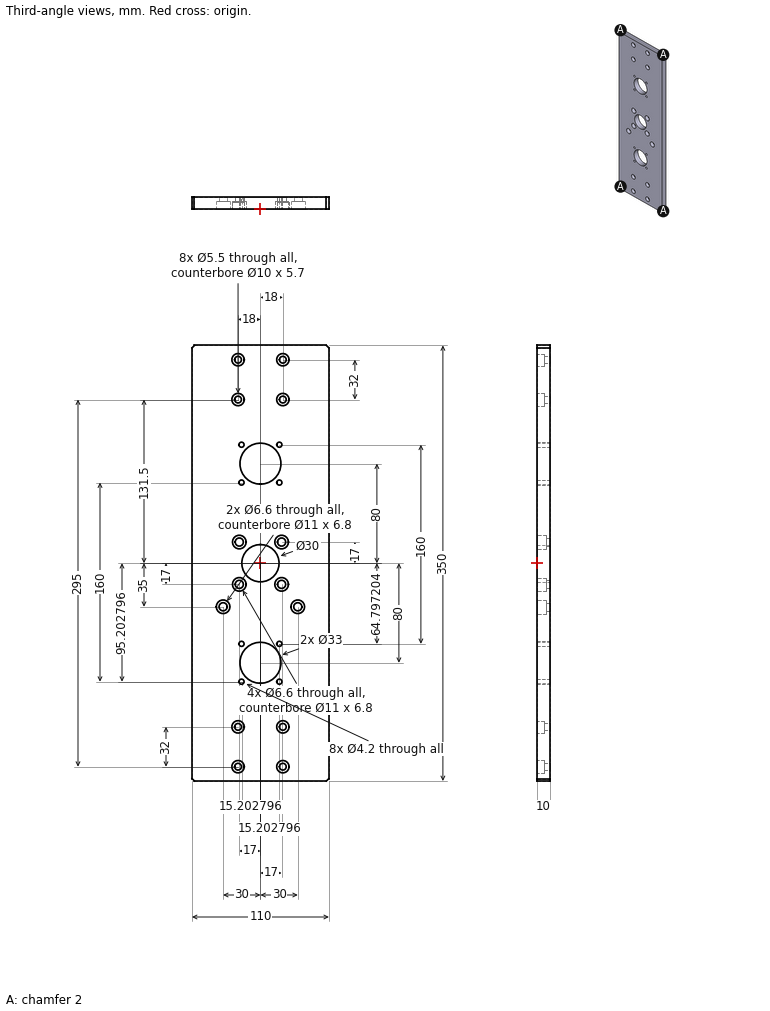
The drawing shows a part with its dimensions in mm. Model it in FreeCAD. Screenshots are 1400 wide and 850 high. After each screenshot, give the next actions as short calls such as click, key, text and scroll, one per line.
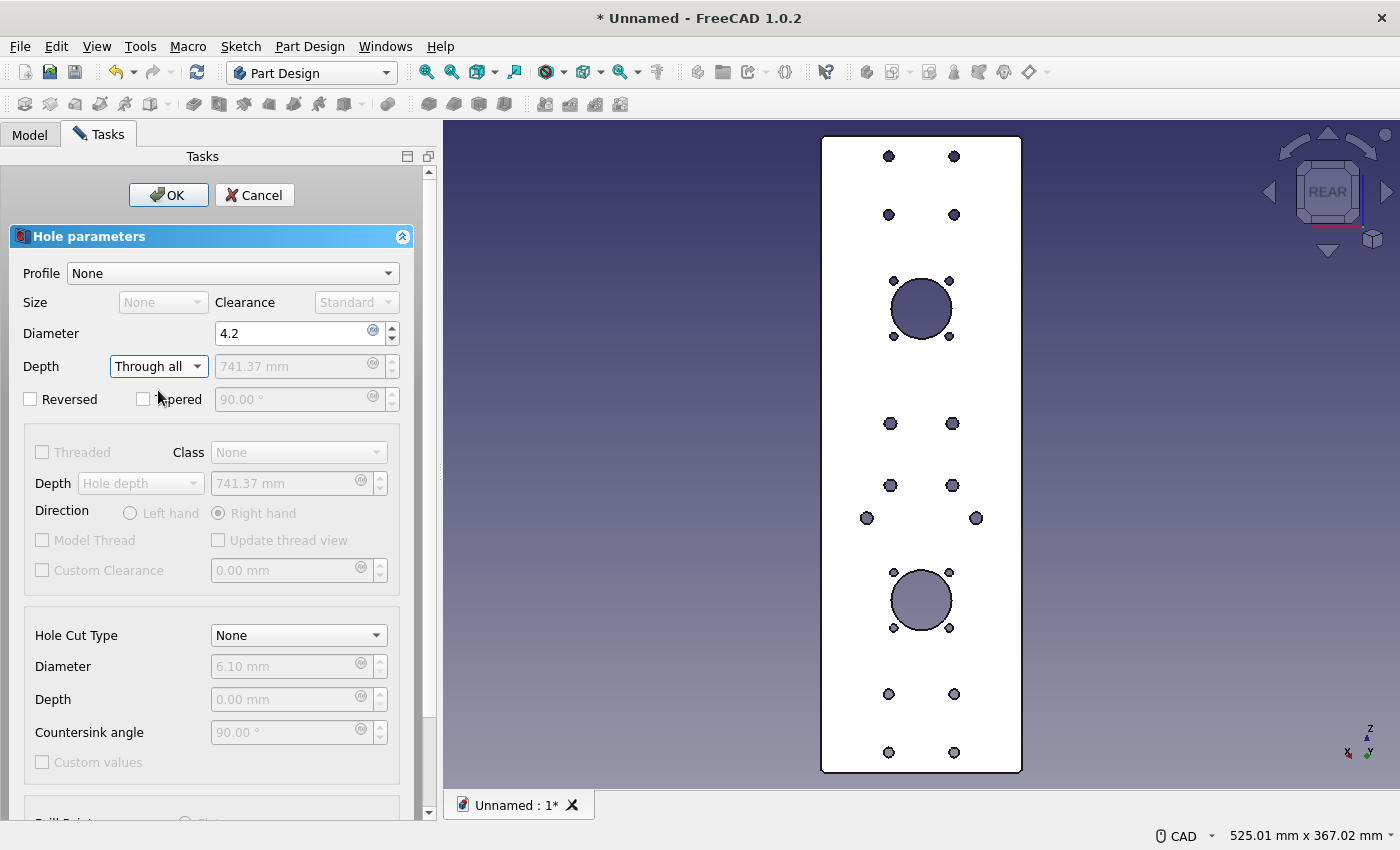
click(169, 195)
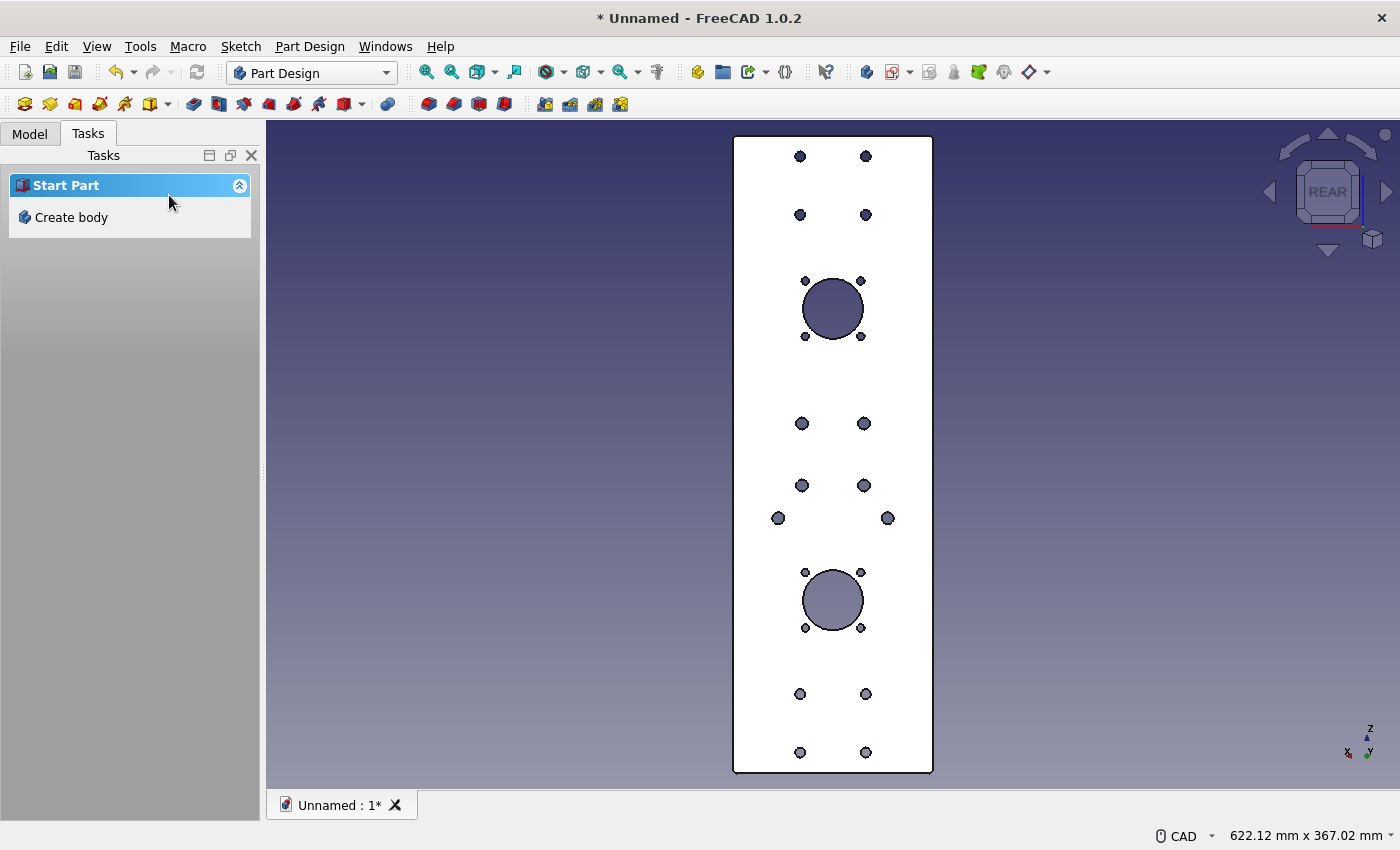
click(833, 454)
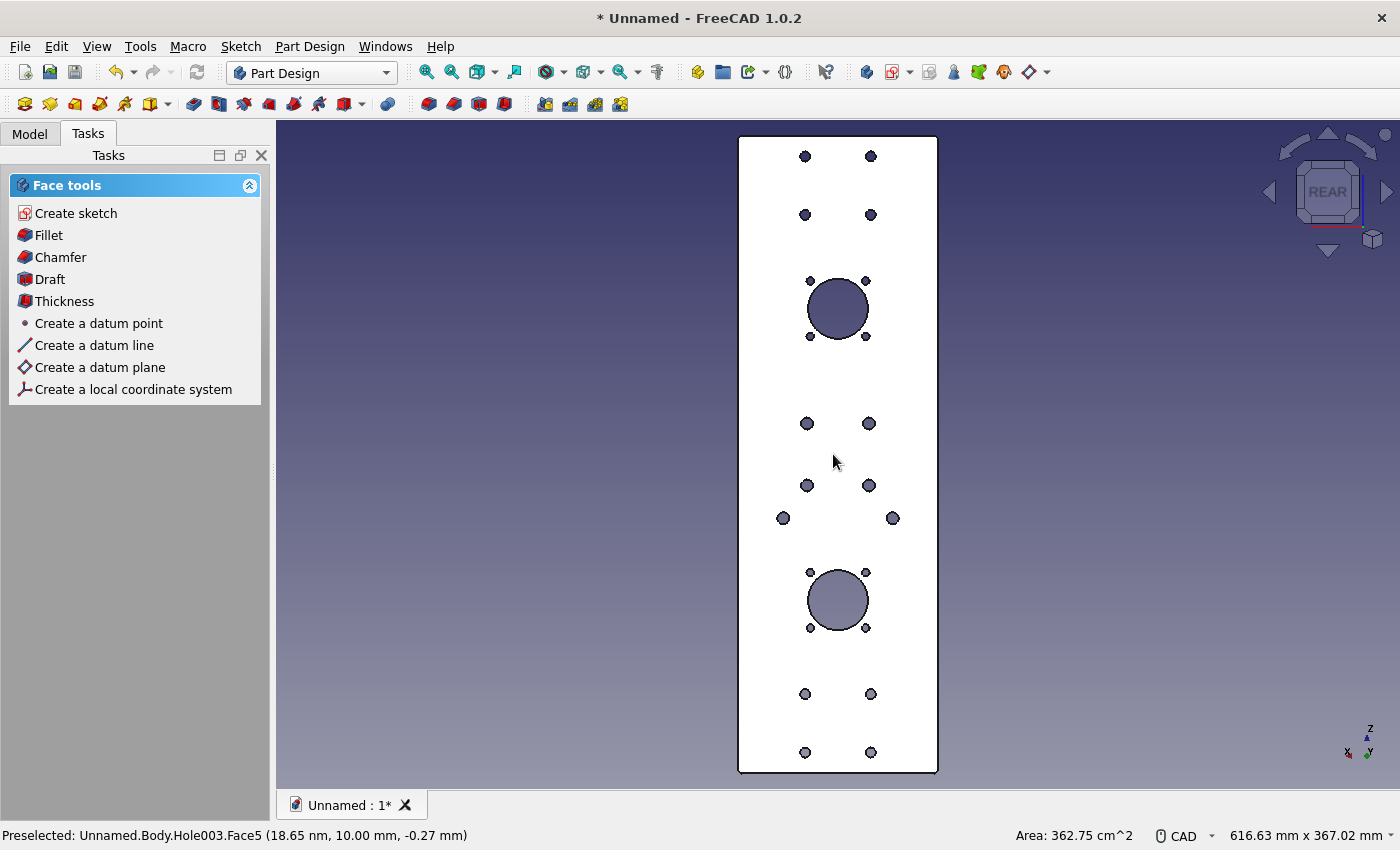
click(892, 72)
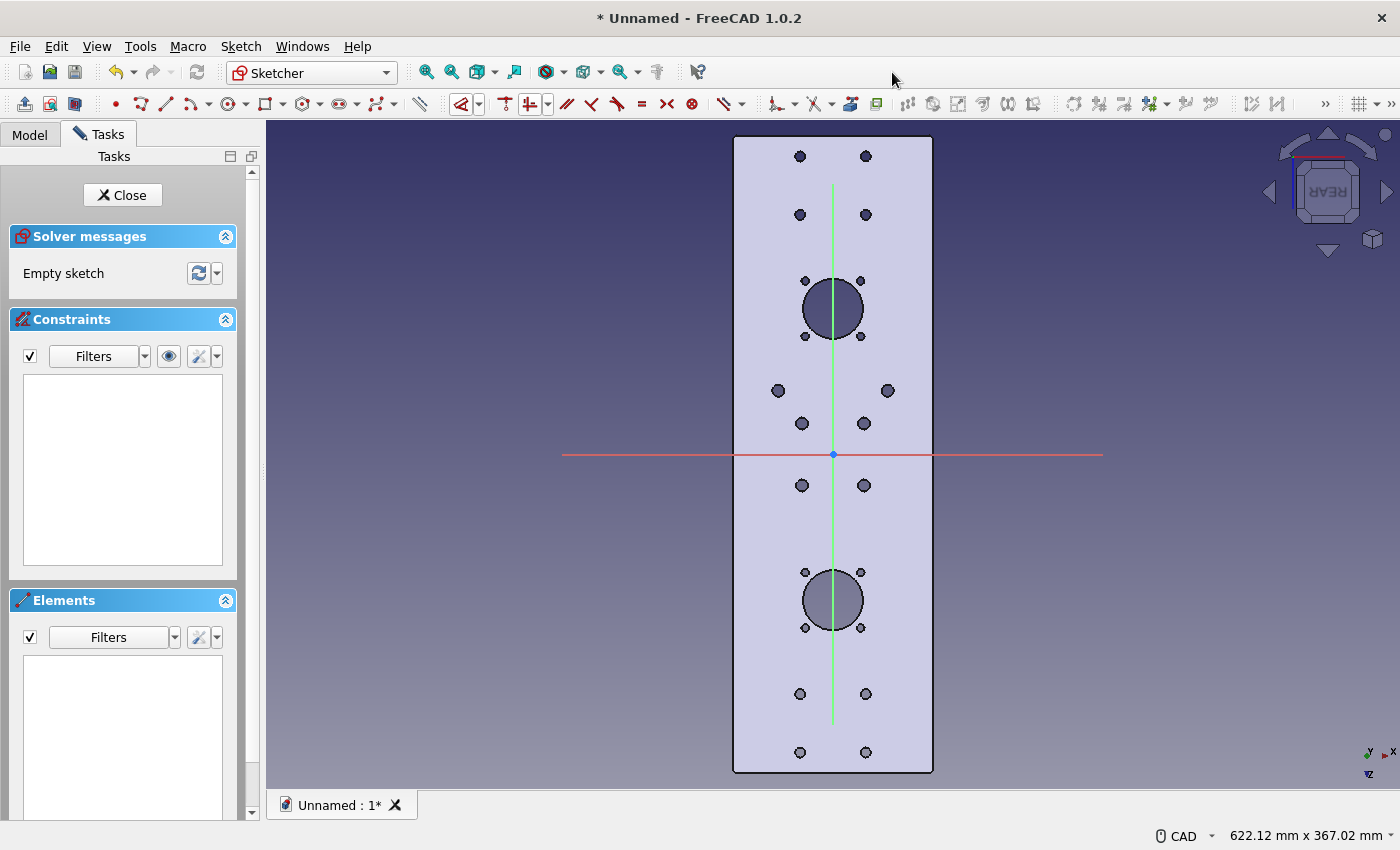
scroll(844, 454, up, 10)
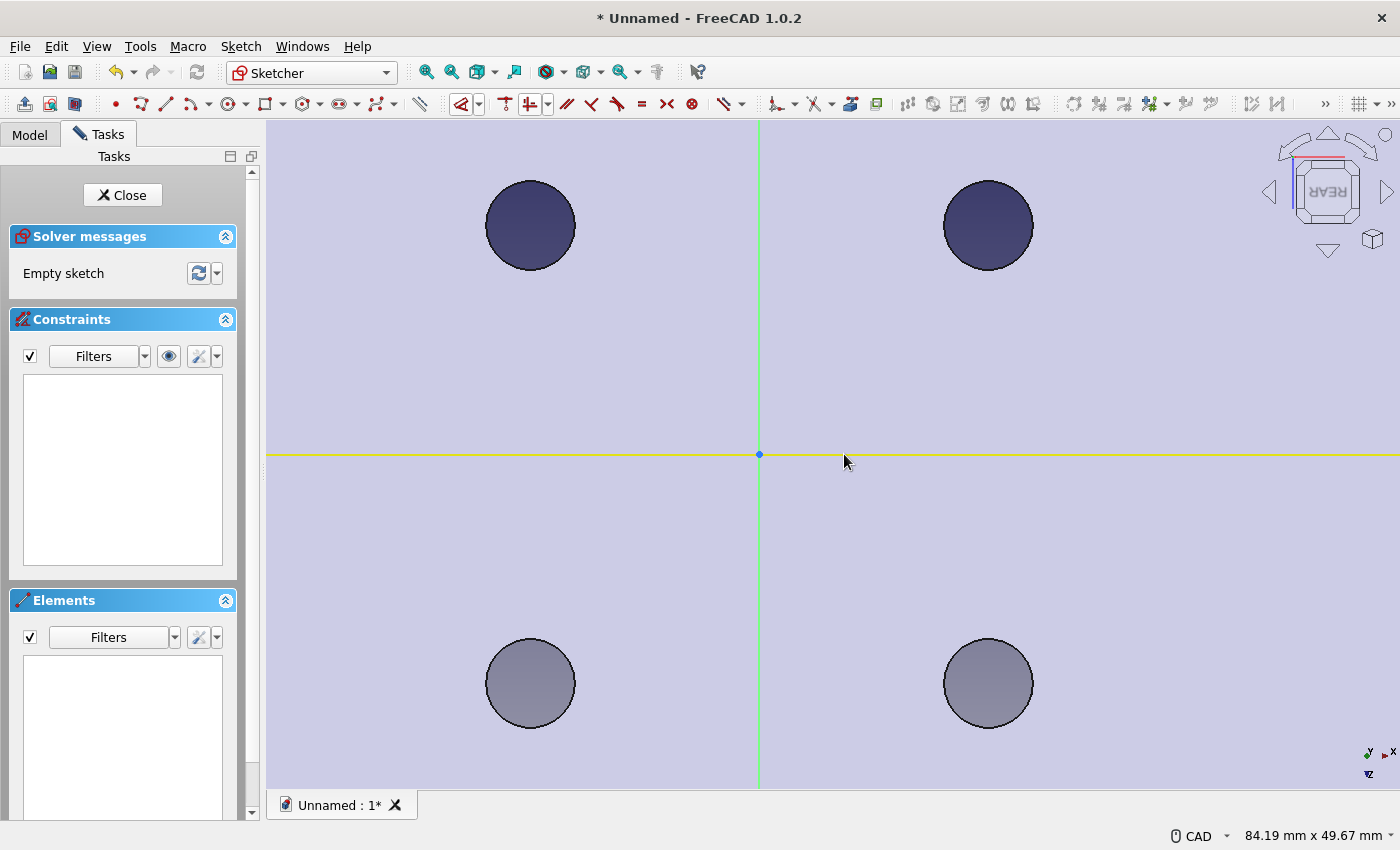
key(g)
key(c)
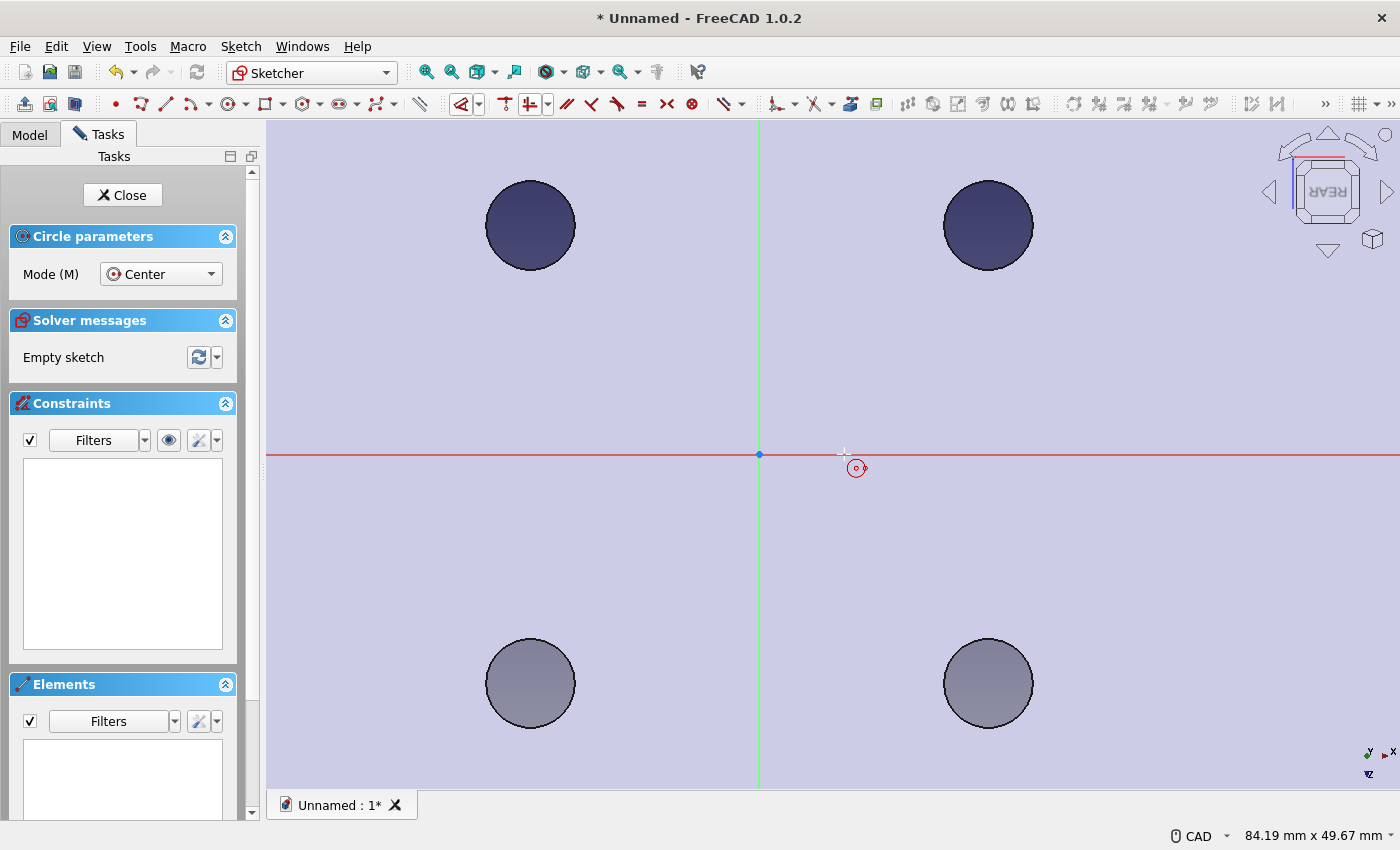
click(759, 454)
move(902, 312)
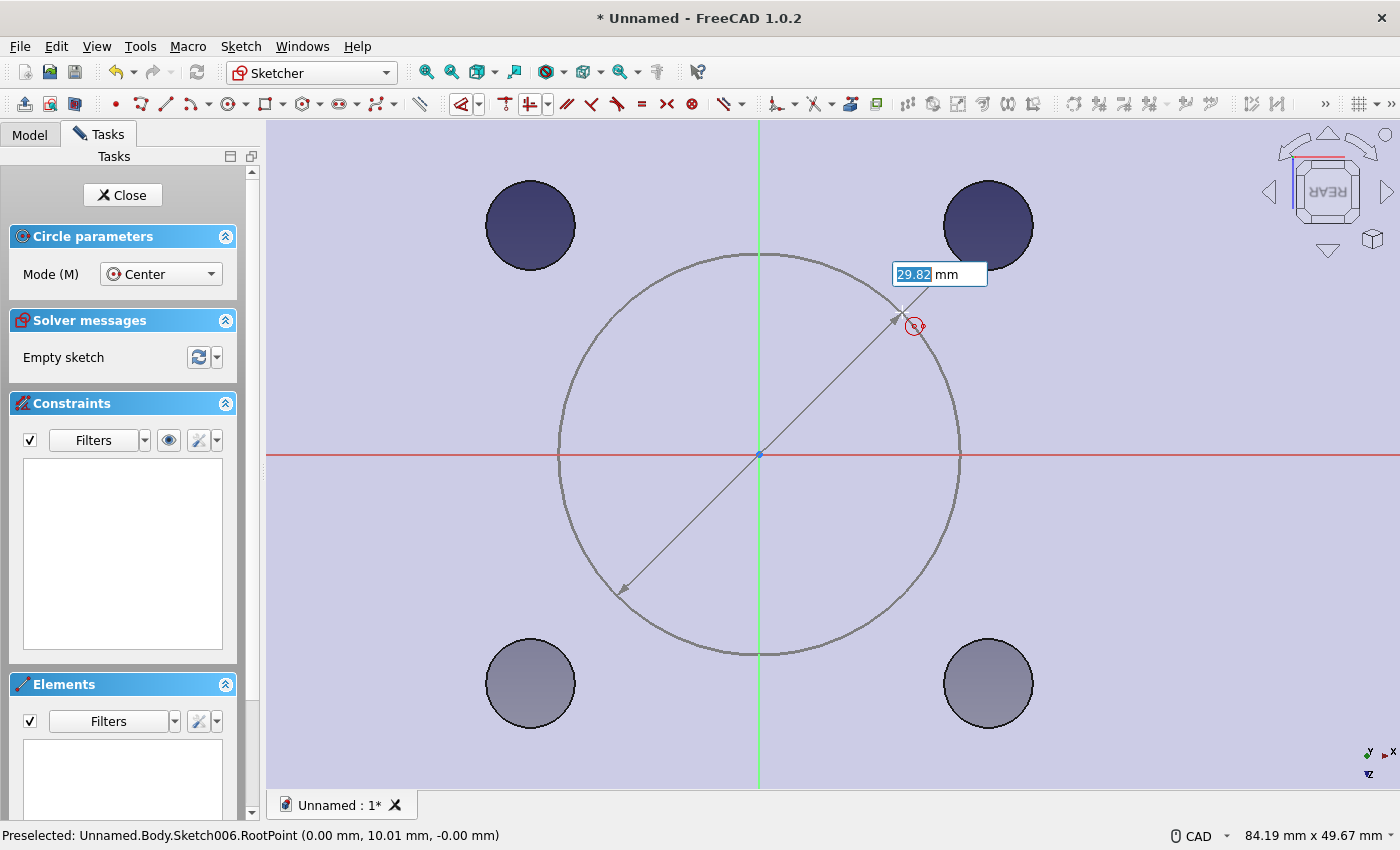
text(30)
key(Return)
key(Escape)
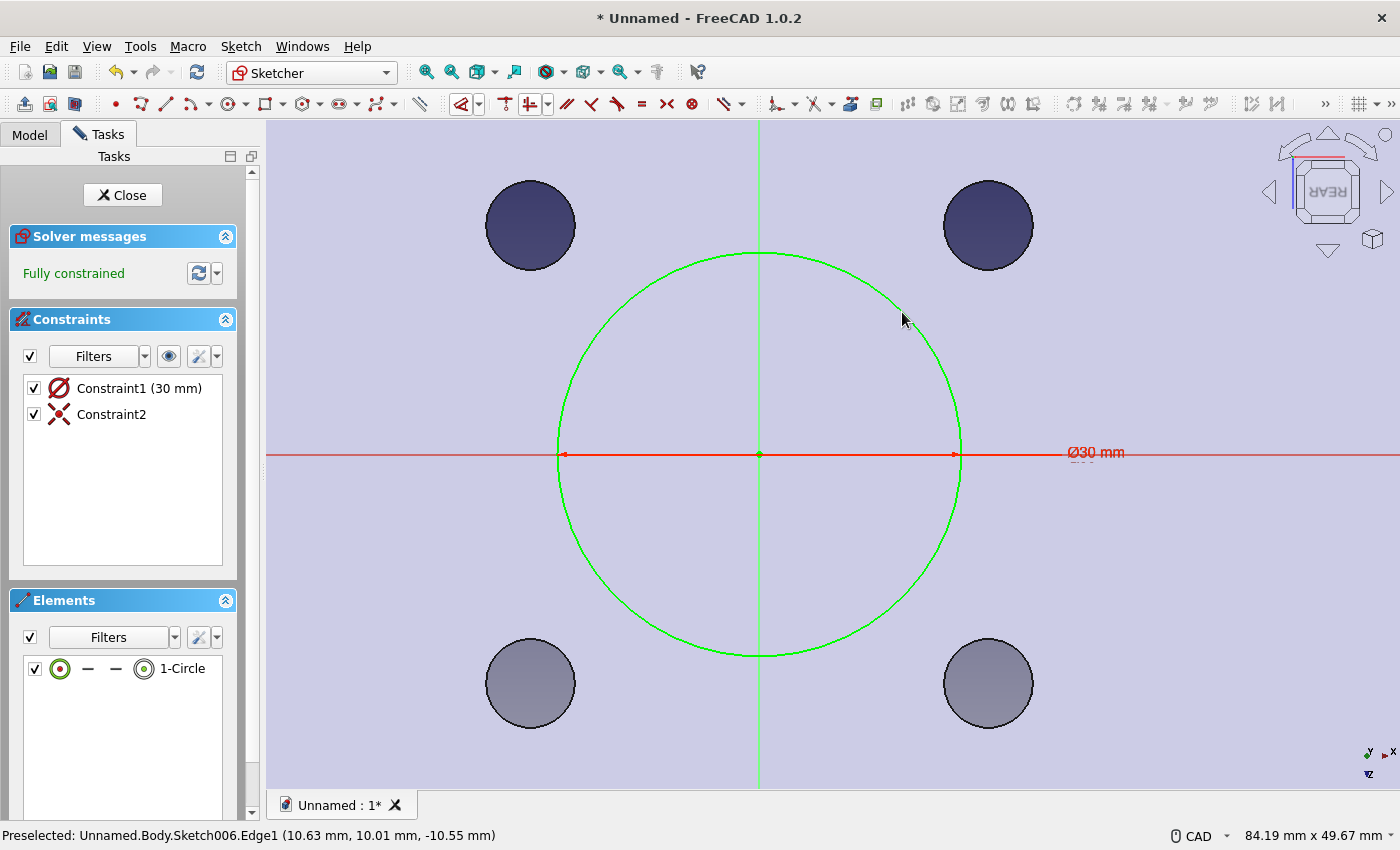
click(123, 195)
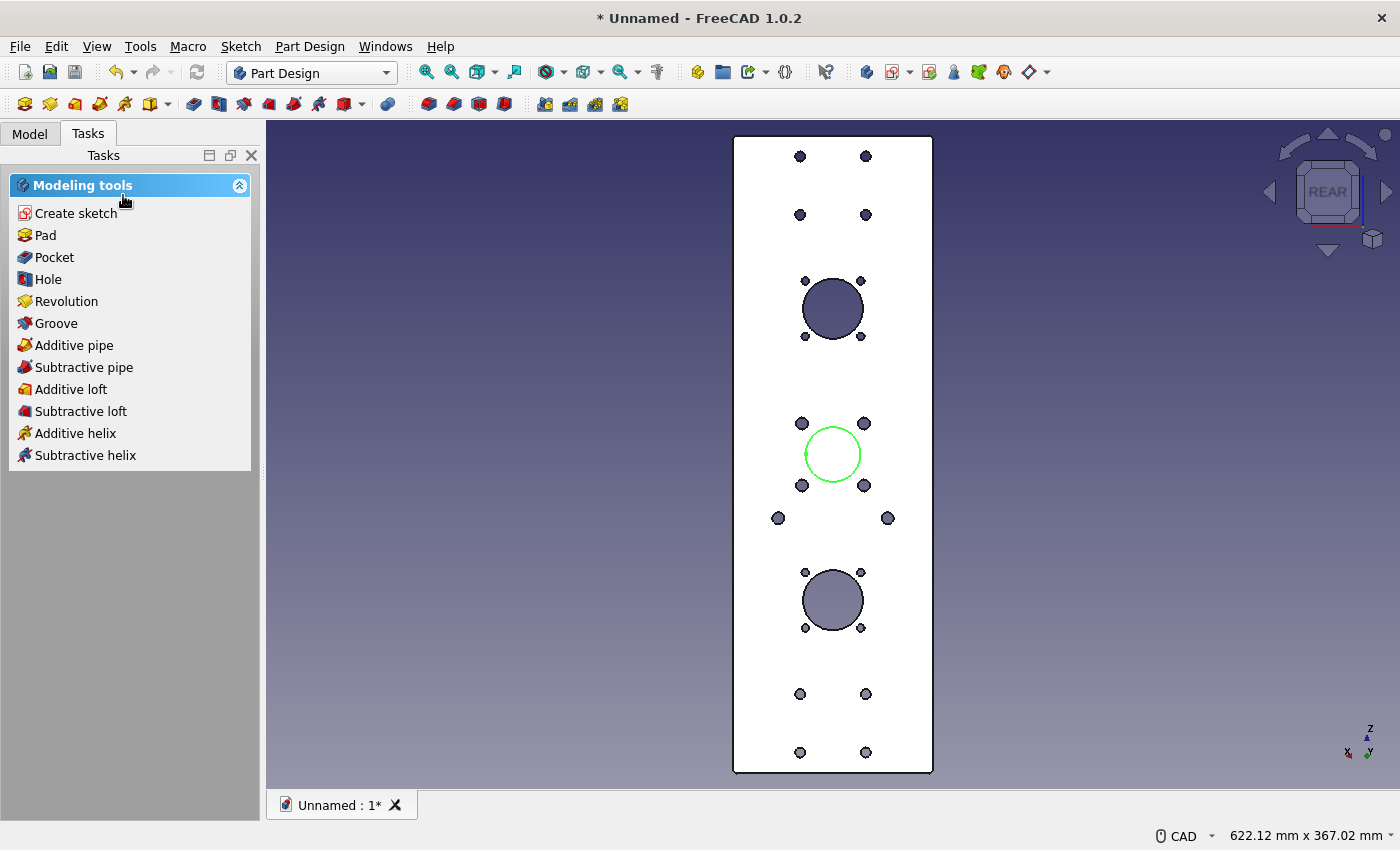
click(194, 104)